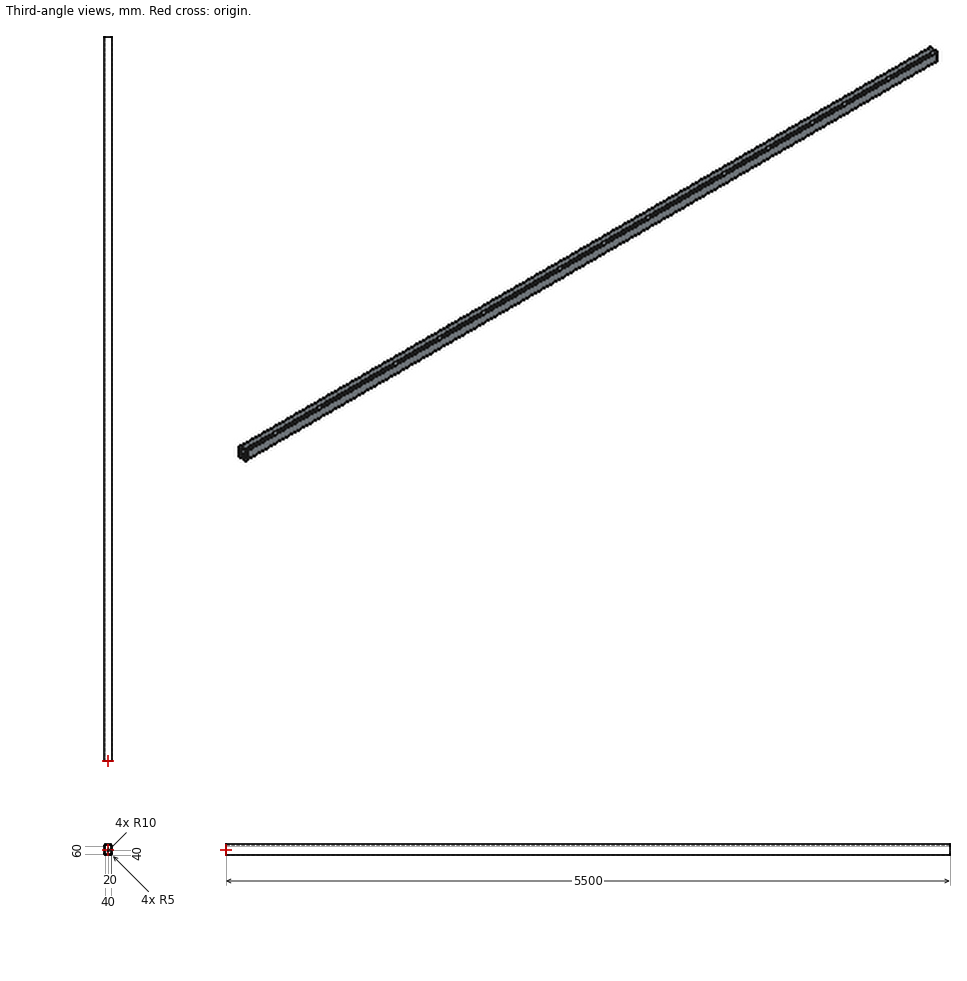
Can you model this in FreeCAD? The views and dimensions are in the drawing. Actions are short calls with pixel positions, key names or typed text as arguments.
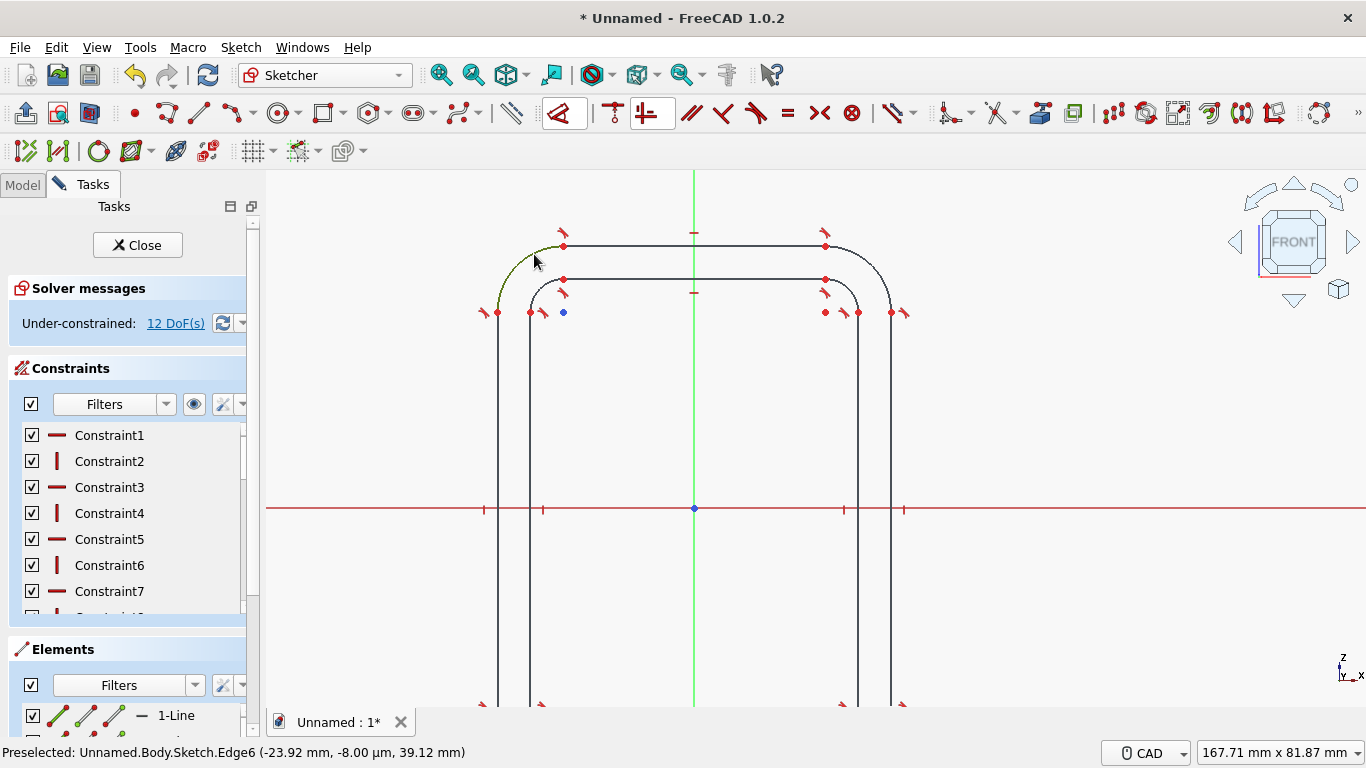
click(549, 283)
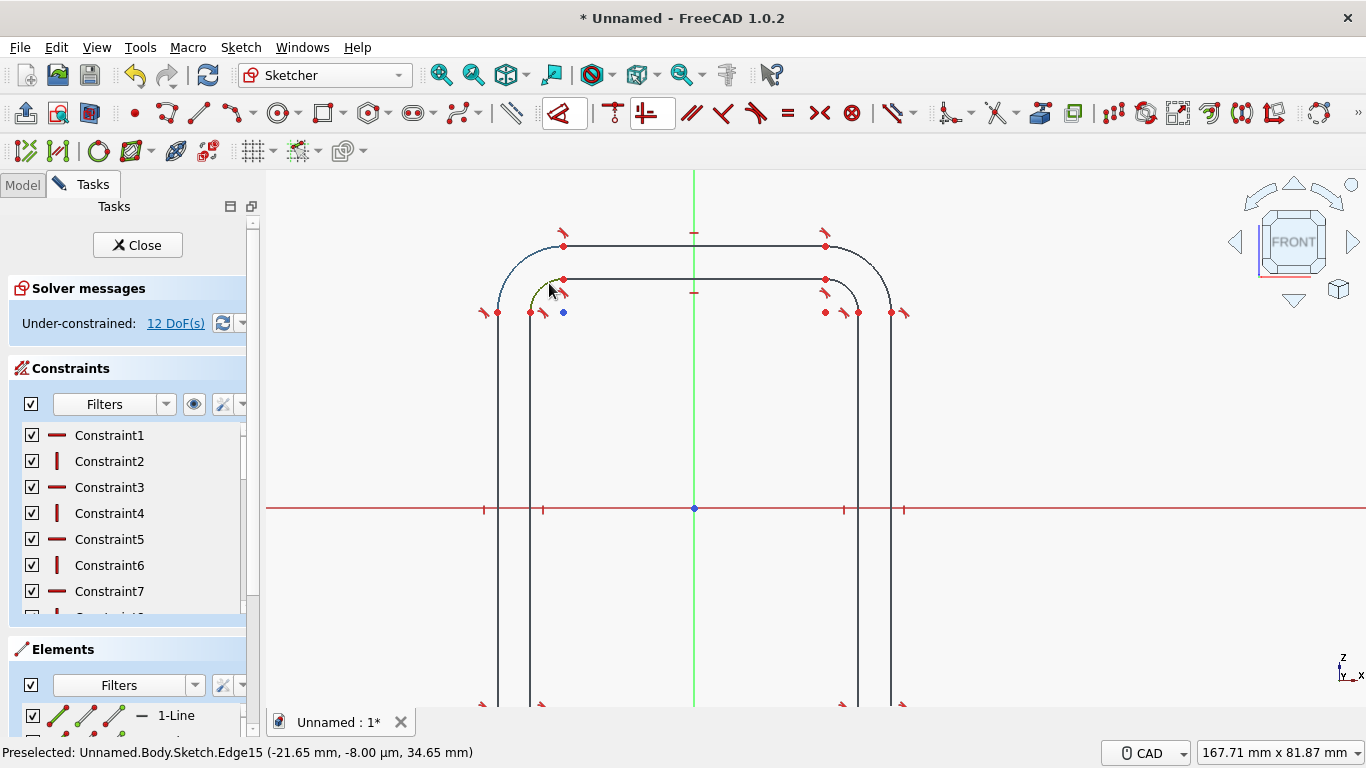
click(614, 114)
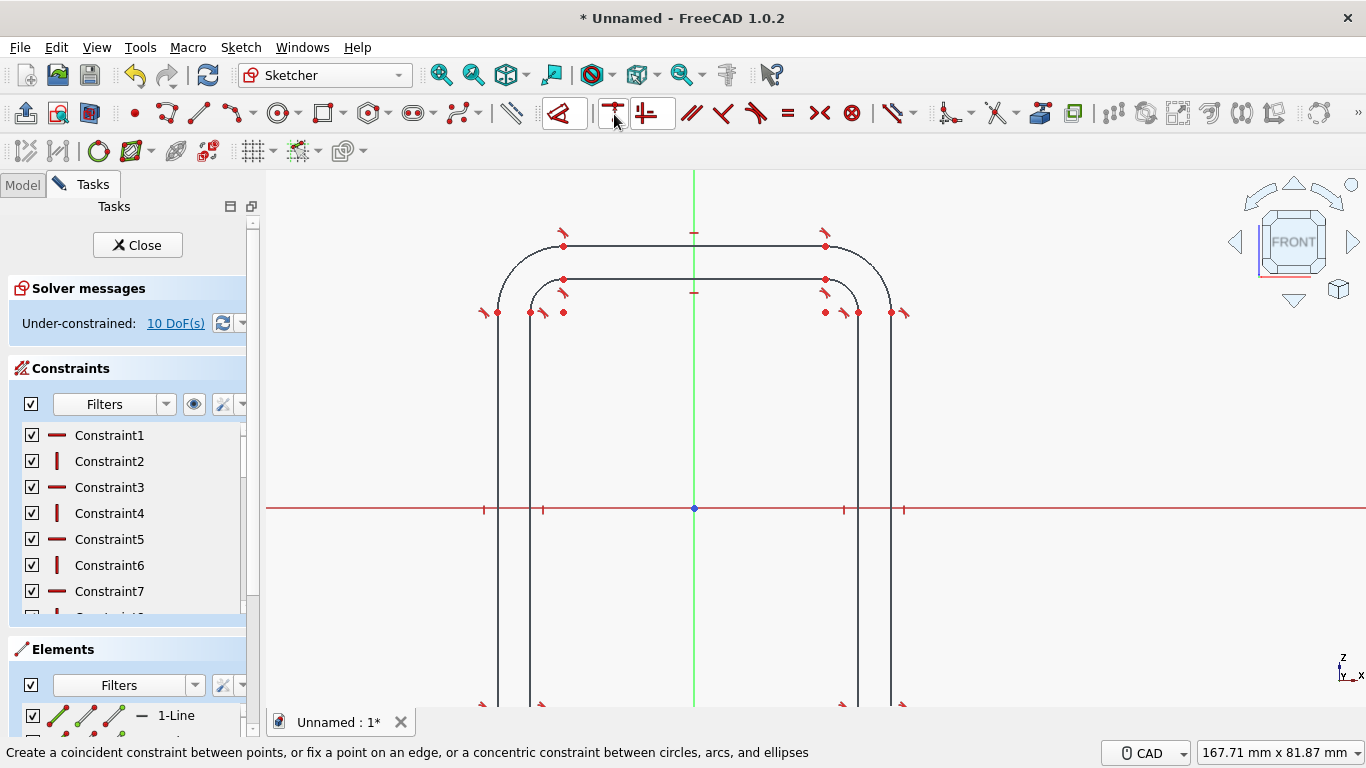
scroll(855, 297, down, 2)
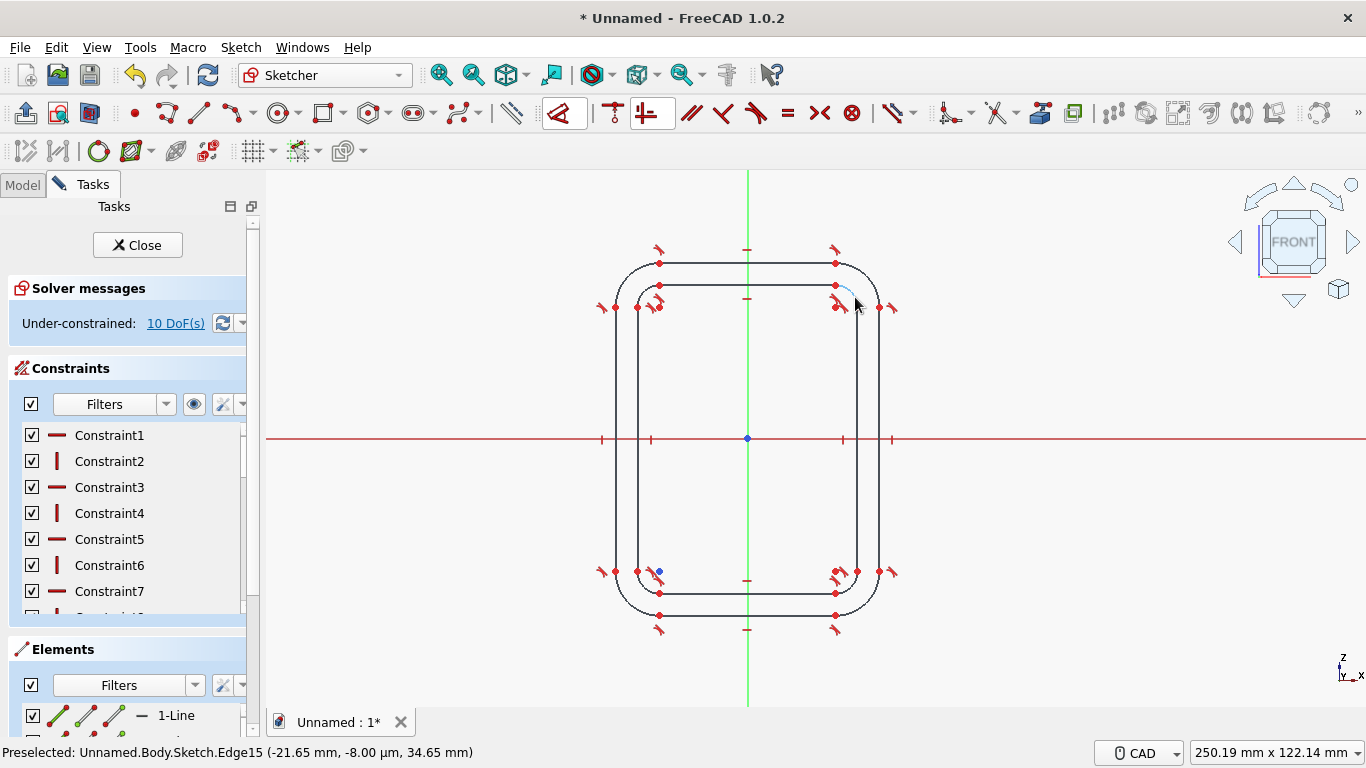
click(620, 592)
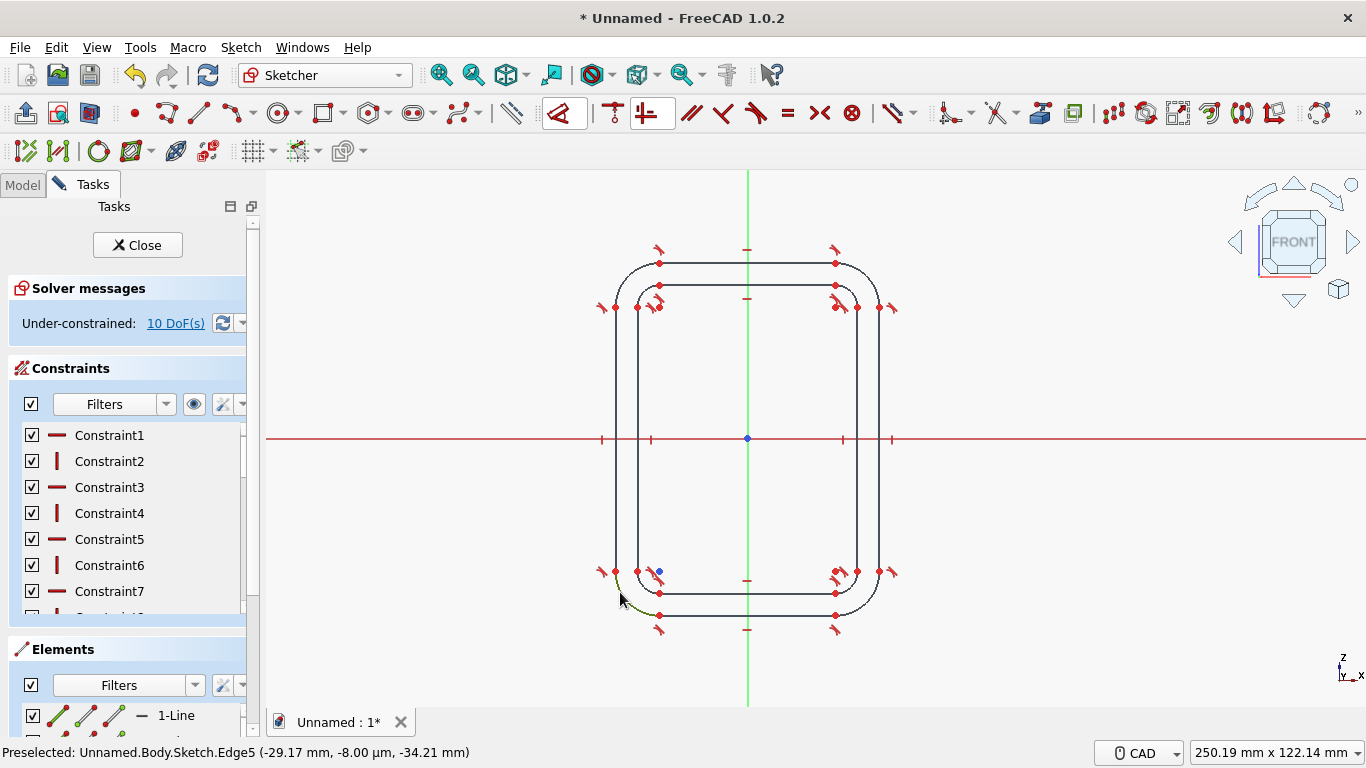
click(640, 268)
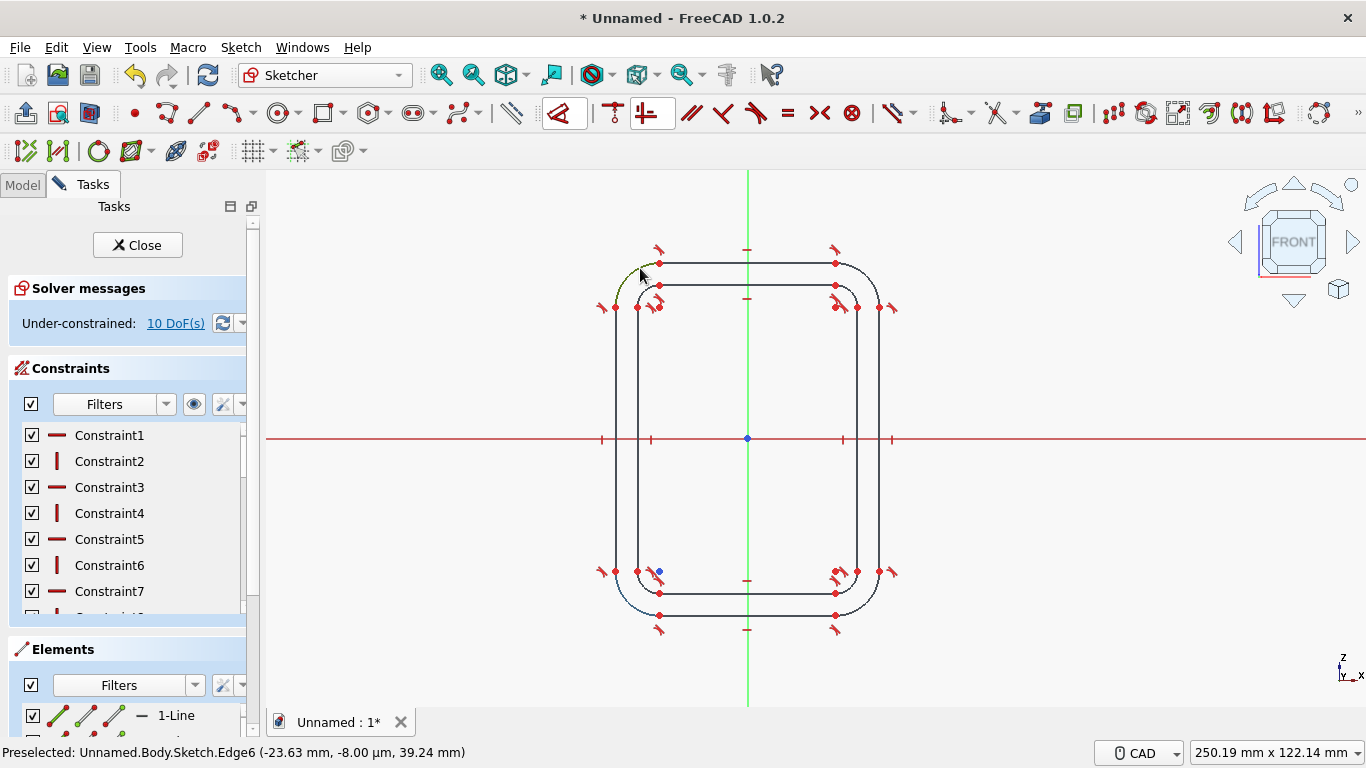
click(875, 287)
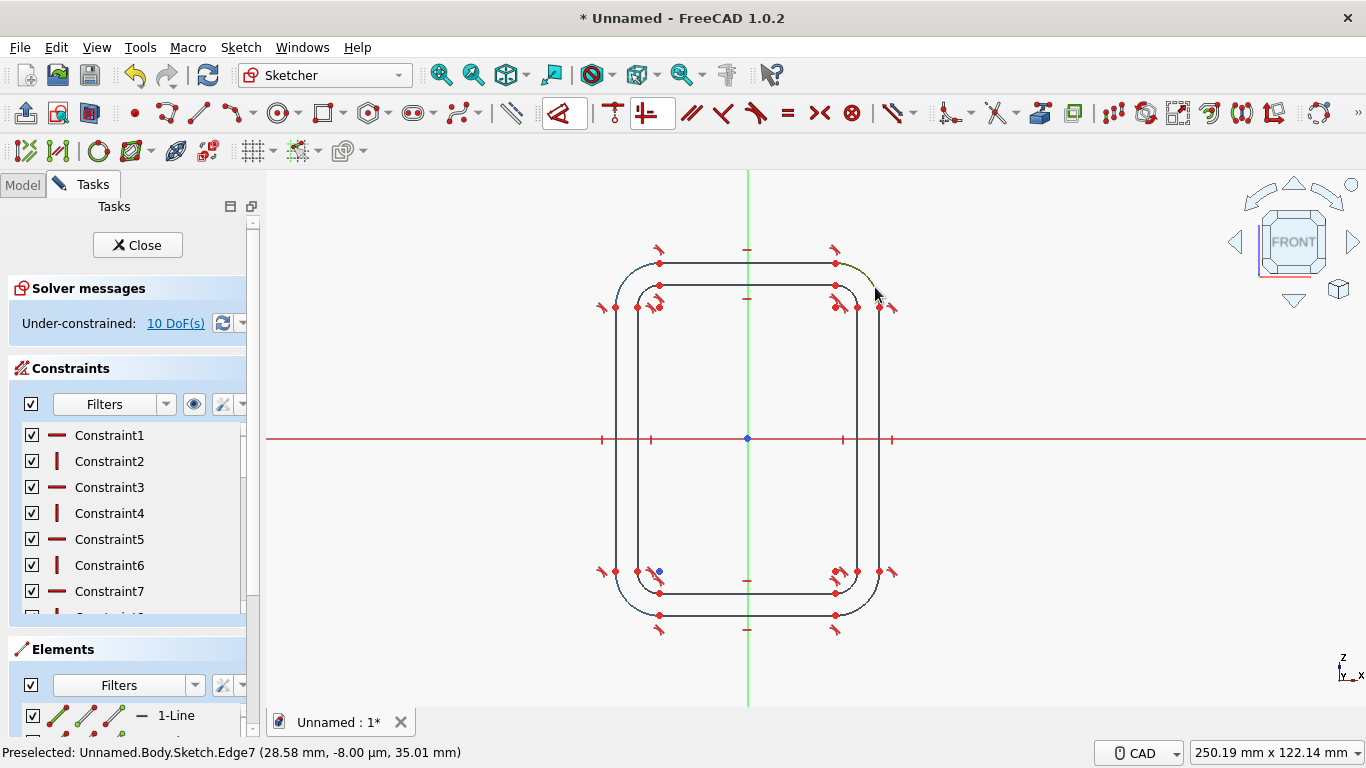
click(855, 611)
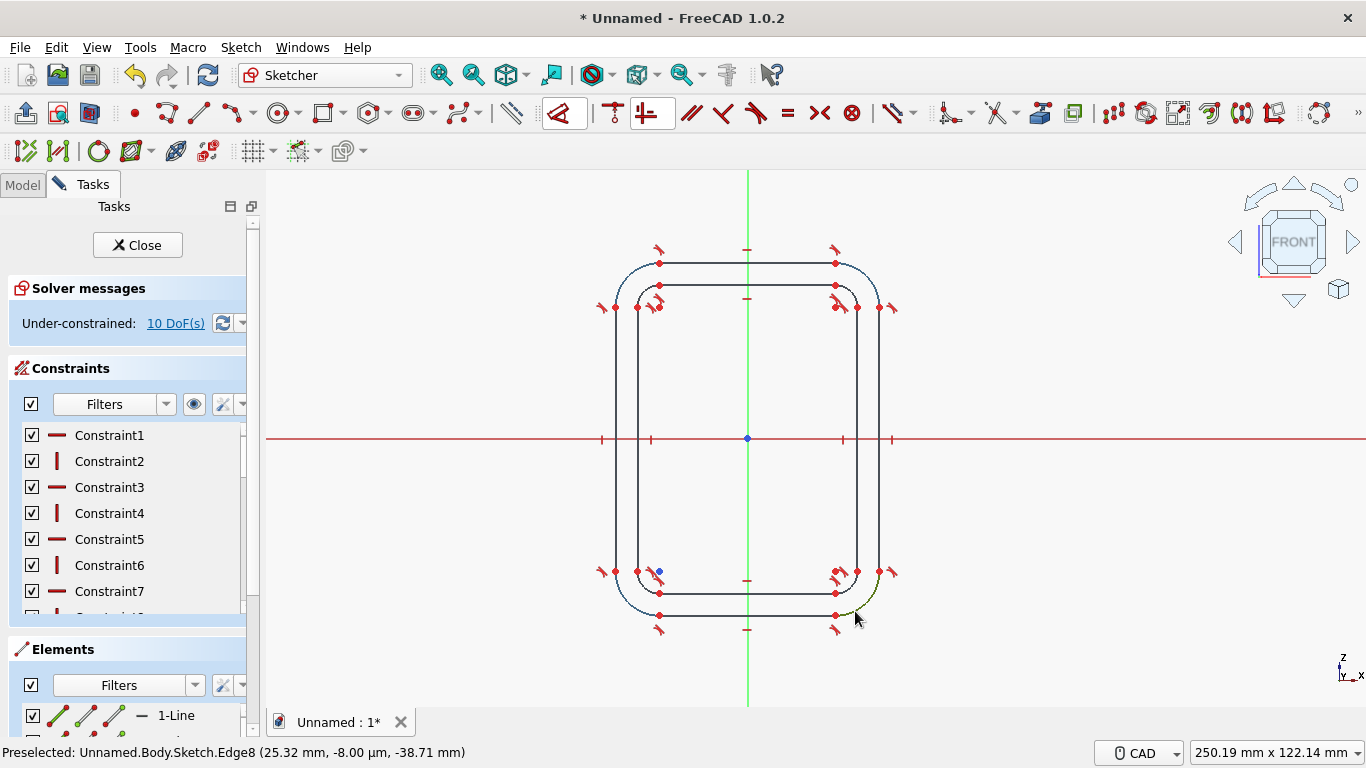
click(788, 114)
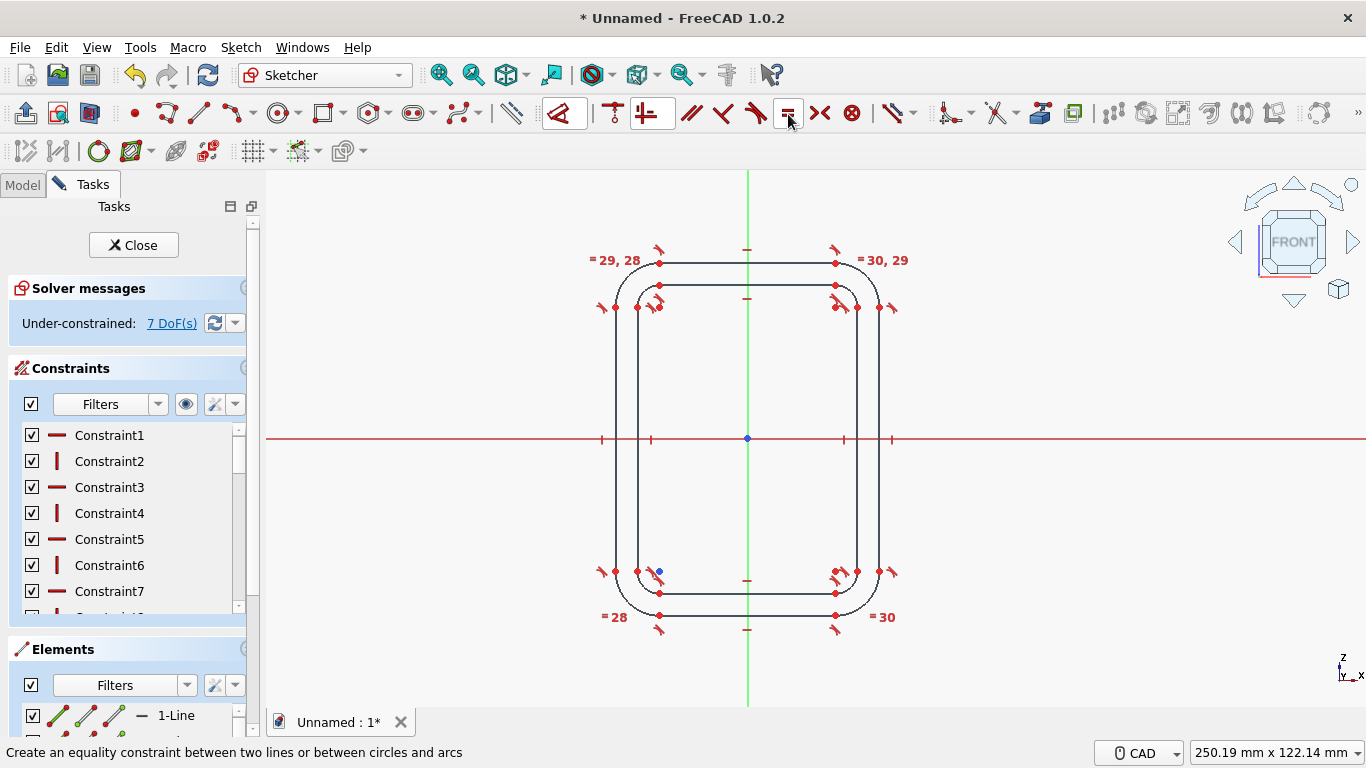
scroll(845, 591, up, 2)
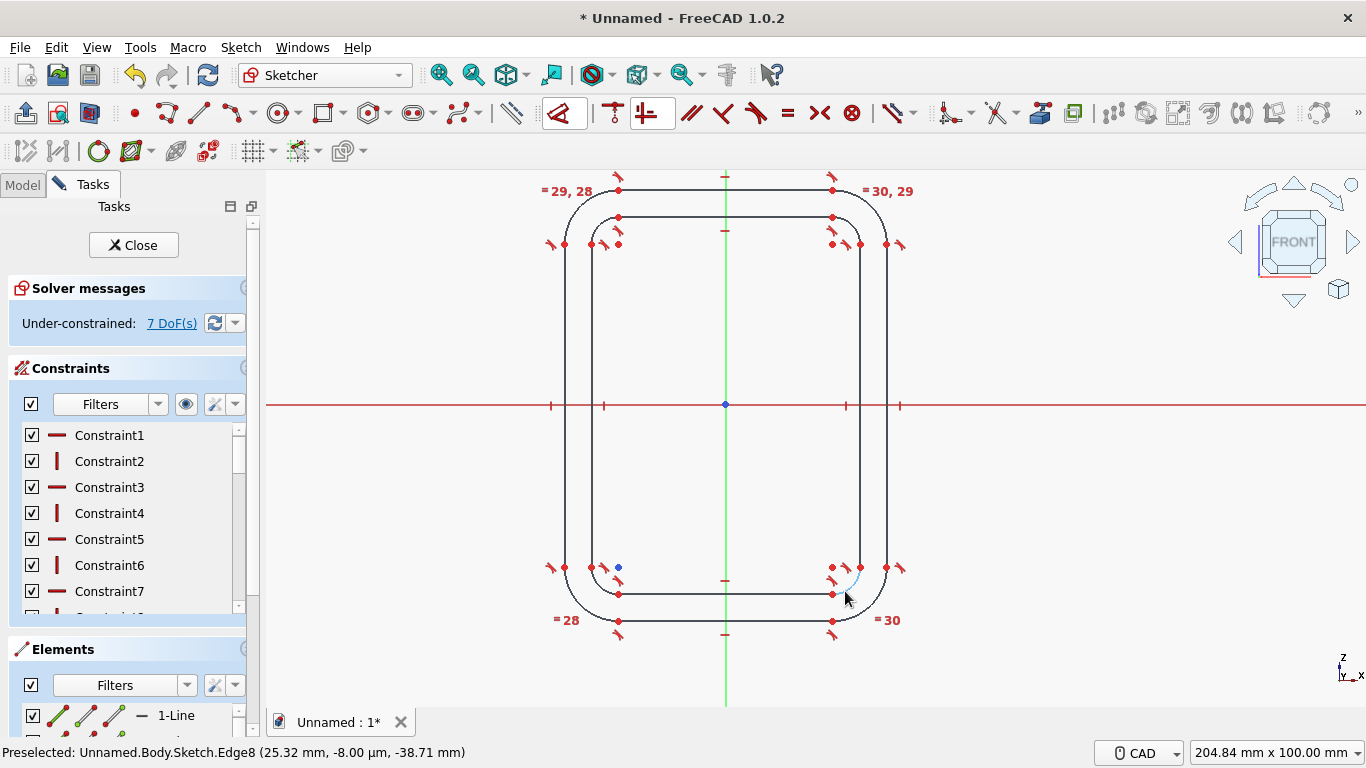
click(845, 591)